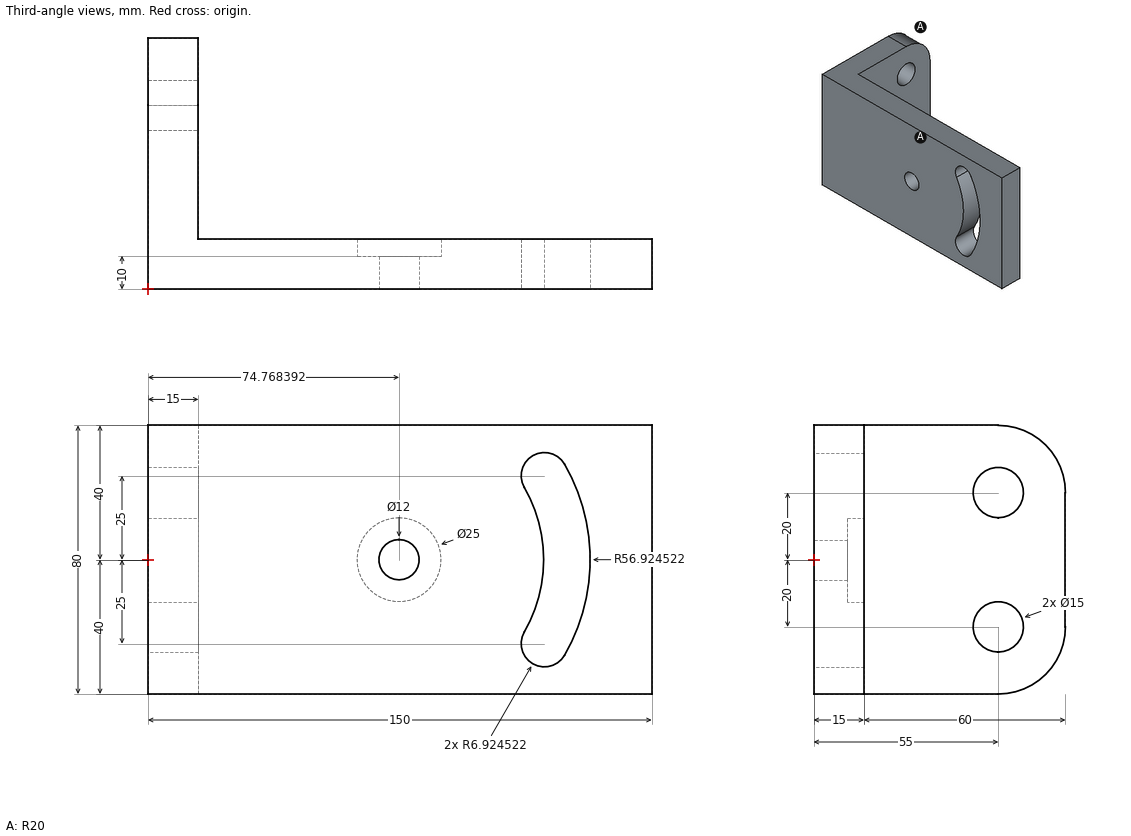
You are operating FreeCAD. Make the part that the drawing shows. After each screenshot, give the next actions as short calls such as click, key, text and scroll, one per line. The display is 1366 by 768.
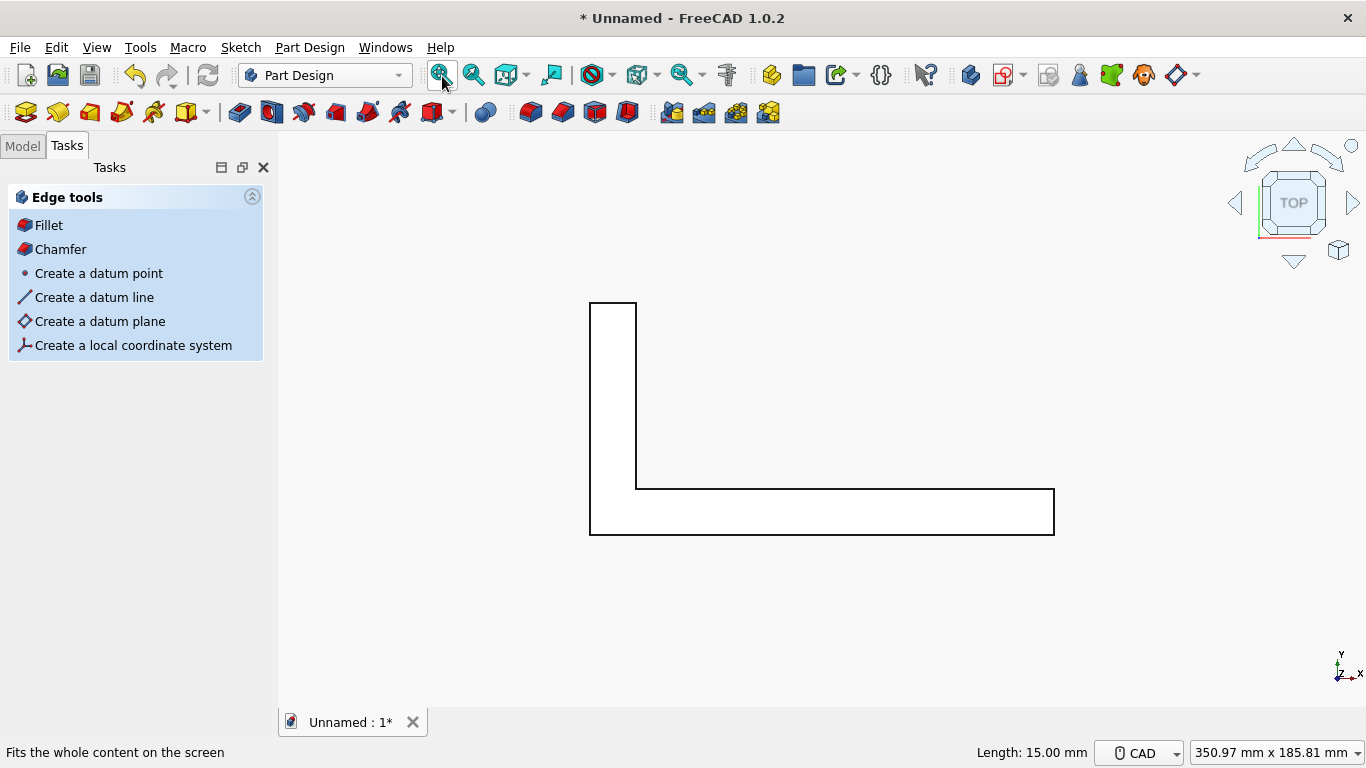
click(613, 302, ctrl)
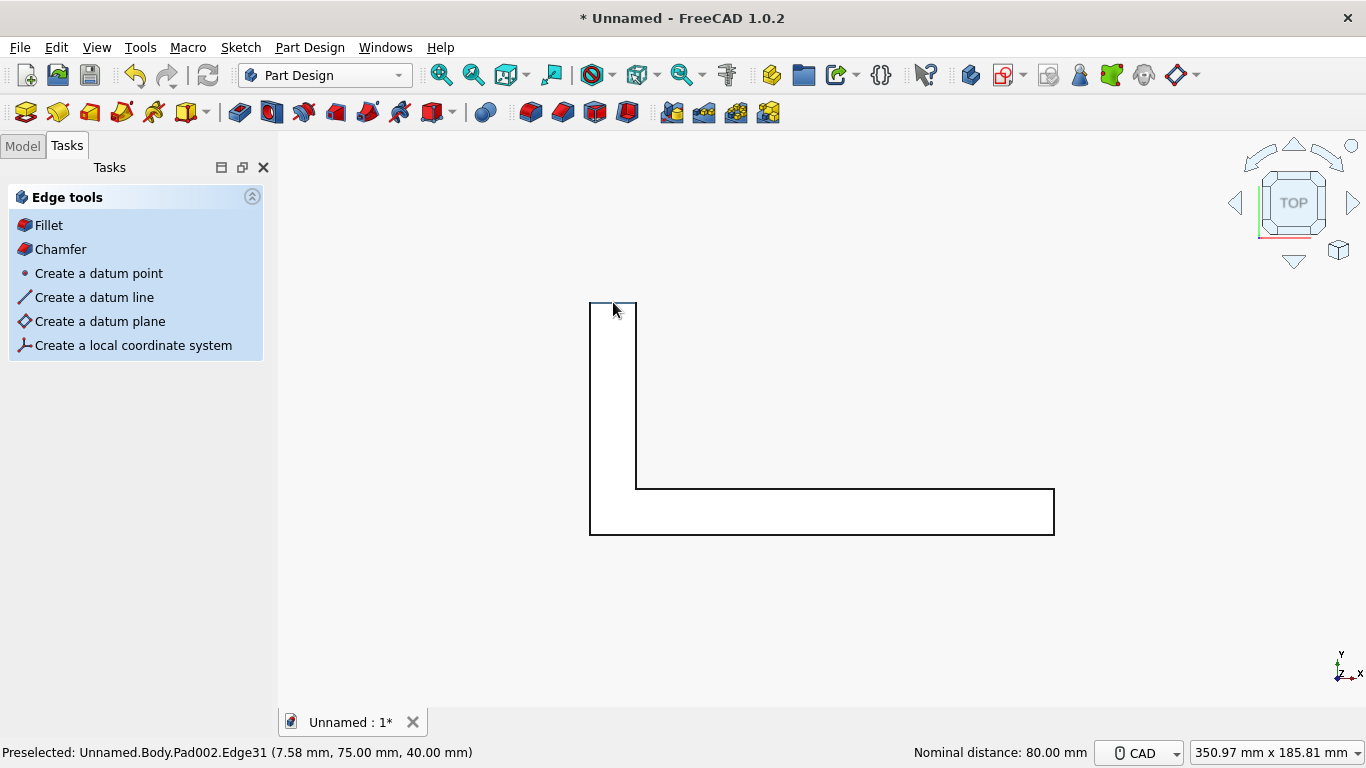
click(532, 112)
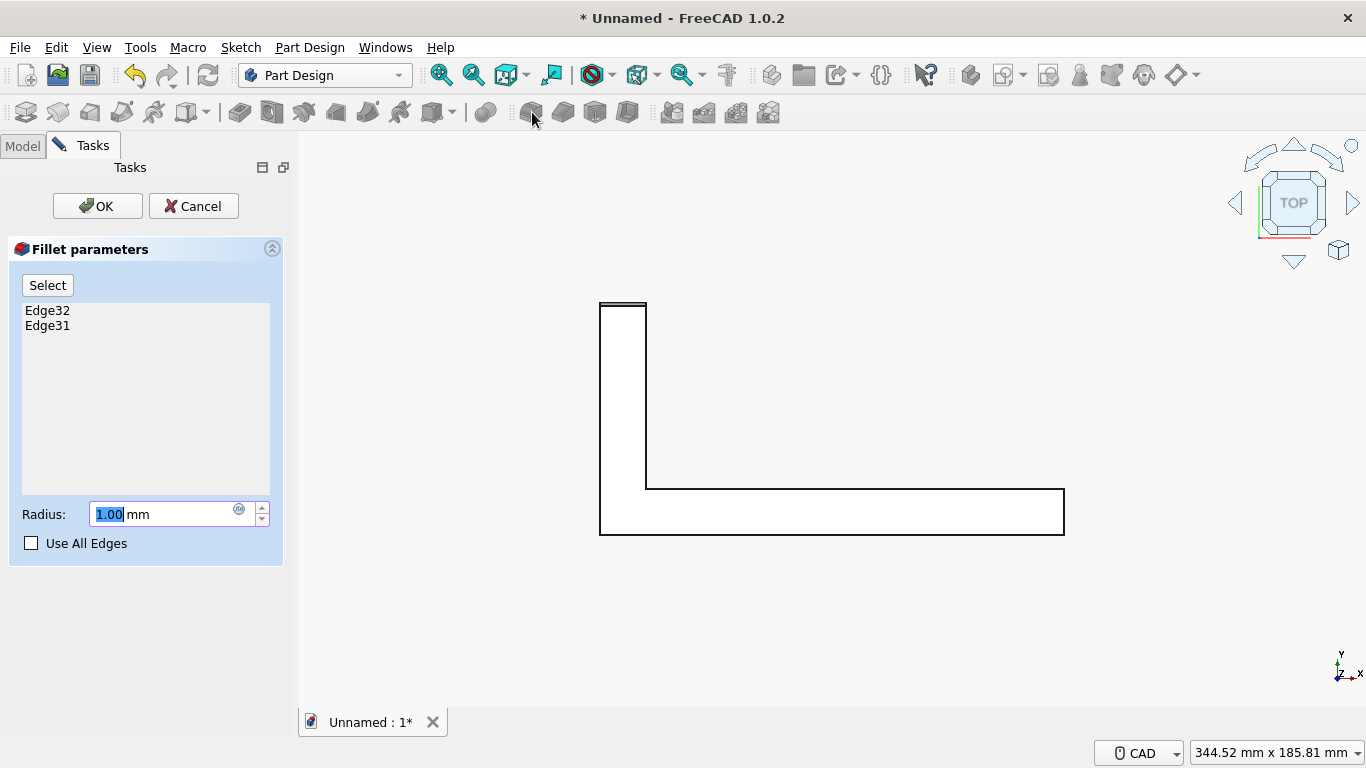
text(20)
key(Tab)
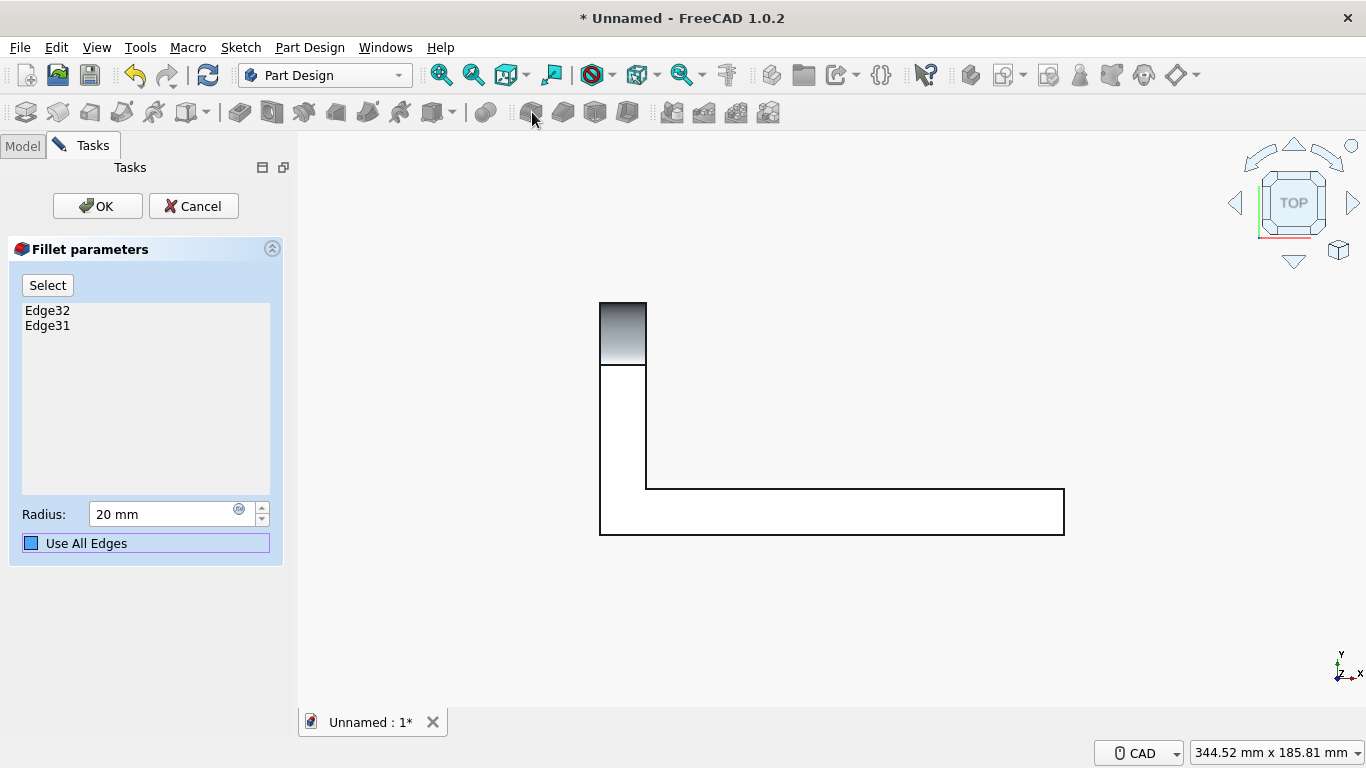
click(98, 206)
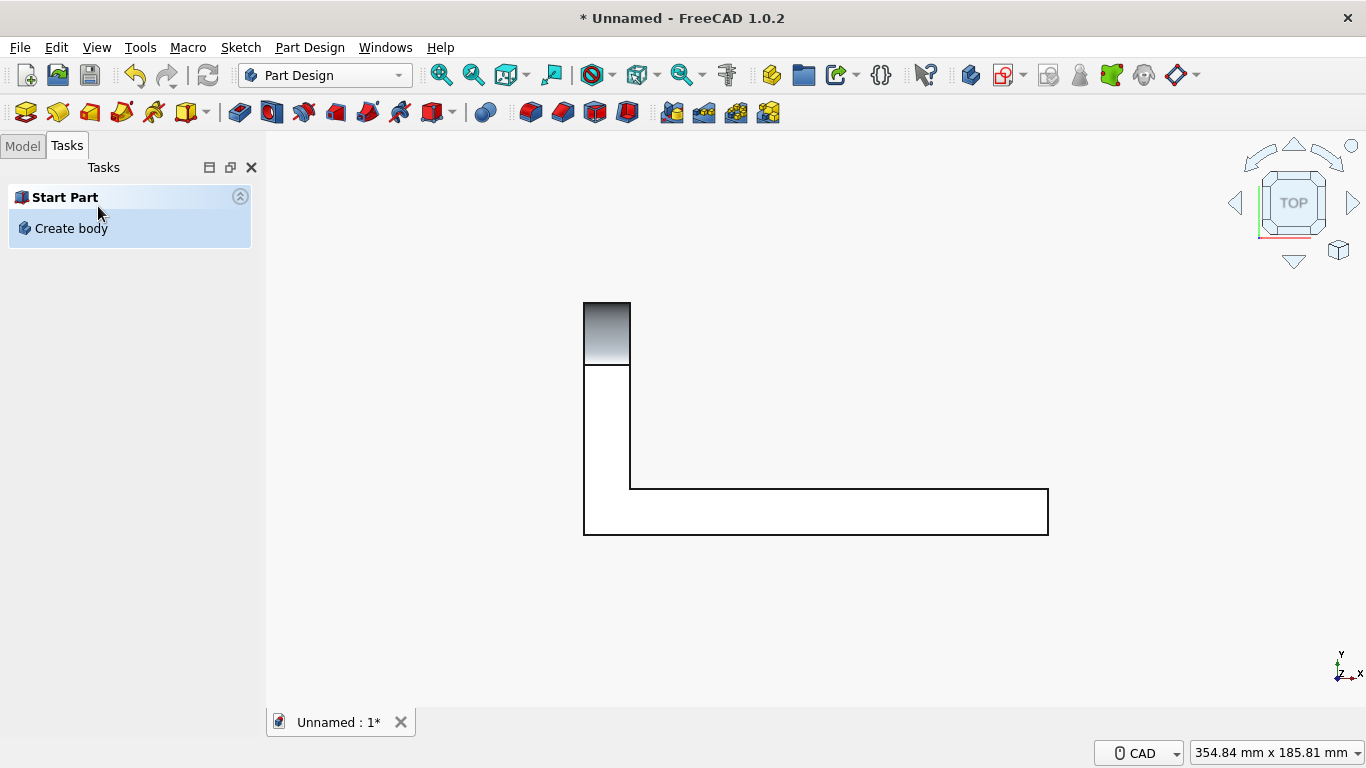
key(v)
key(f)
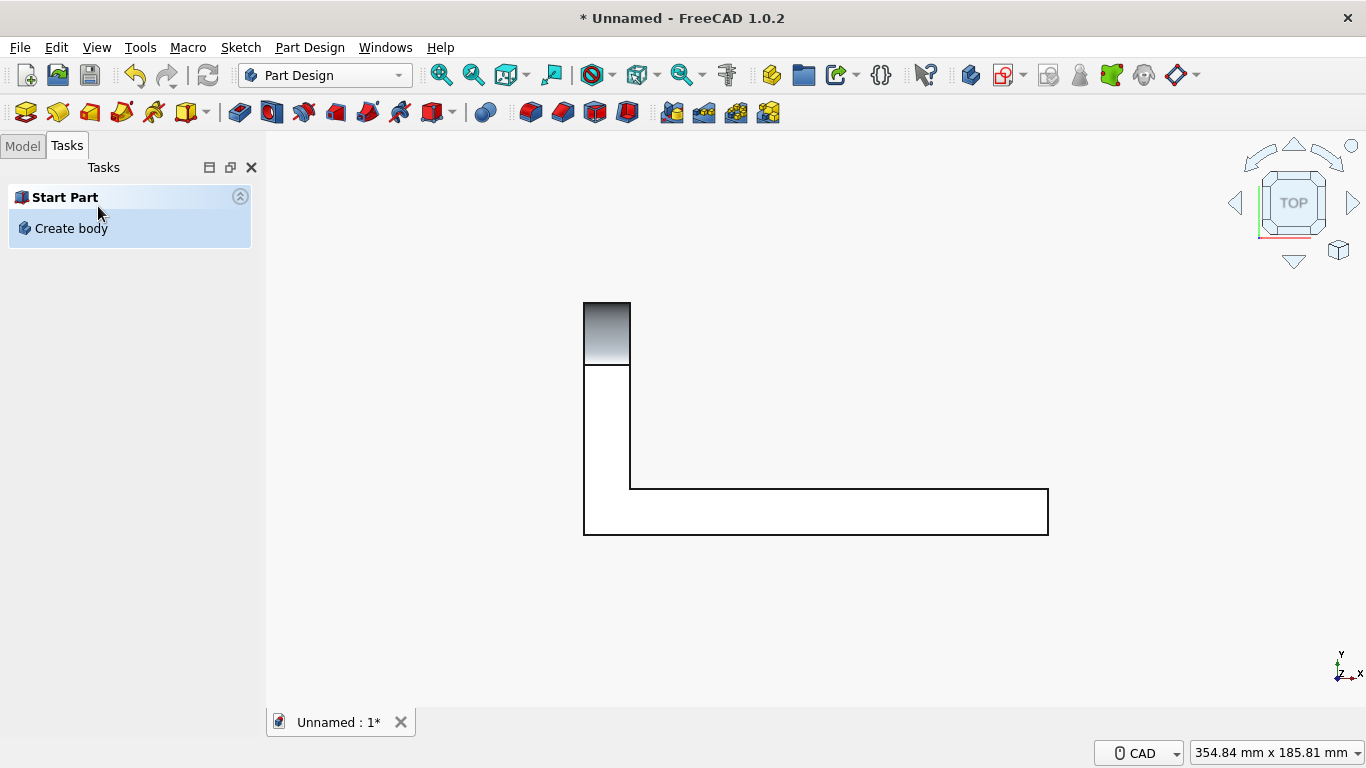
key(0)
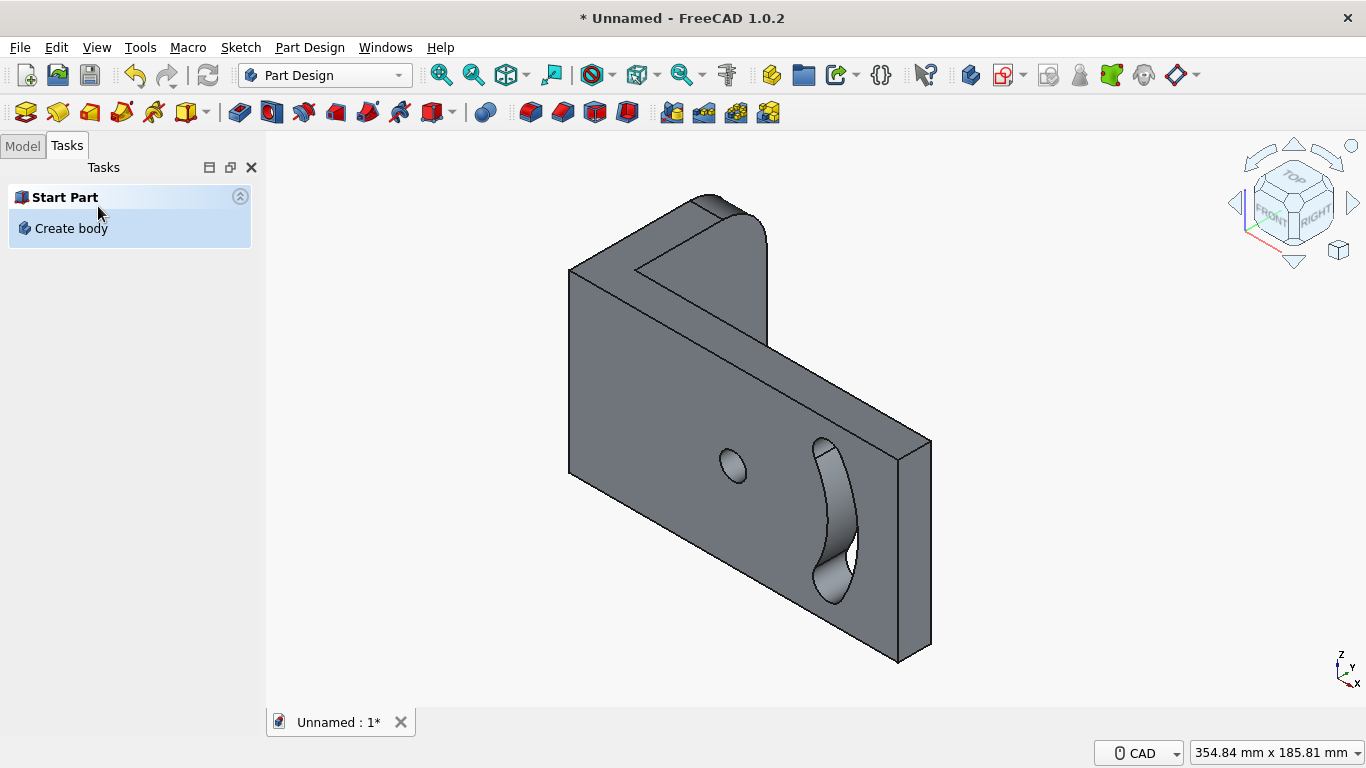
key(3)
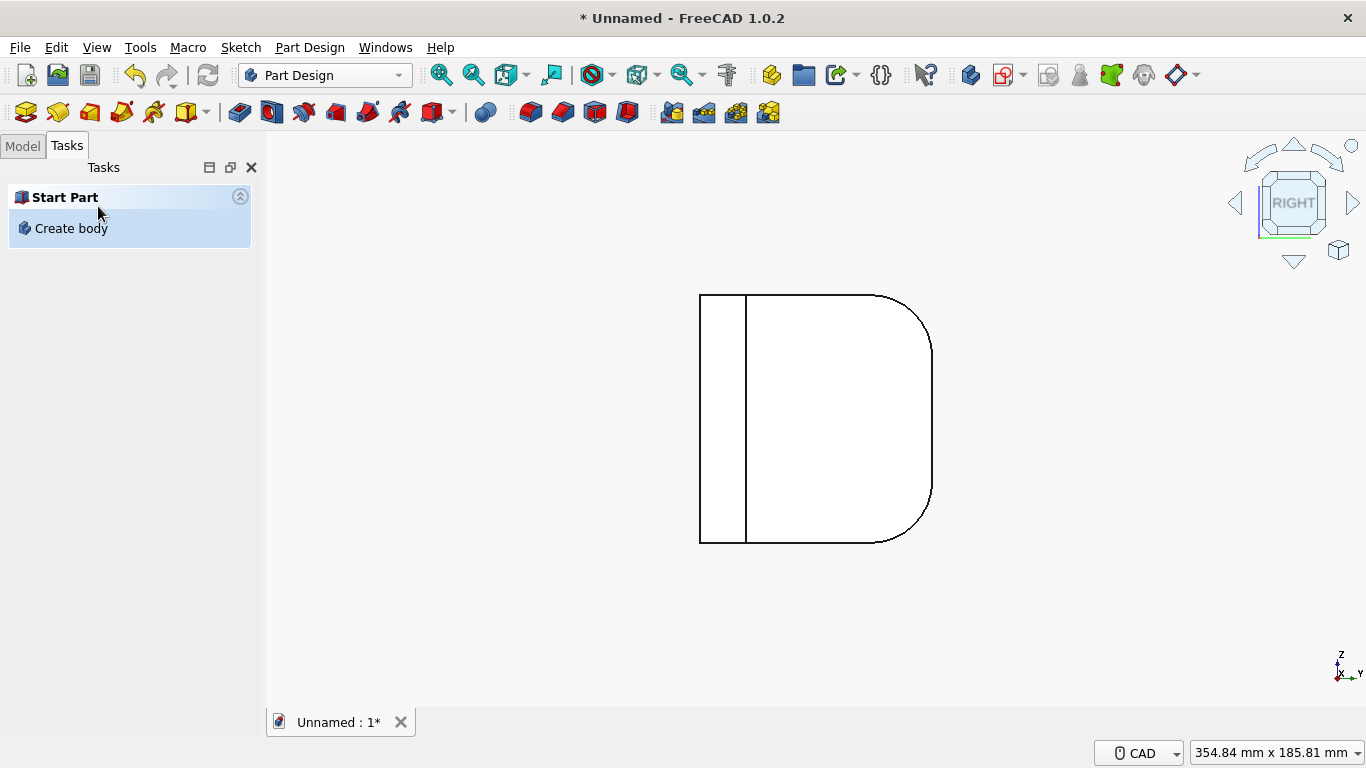
click(442, 76)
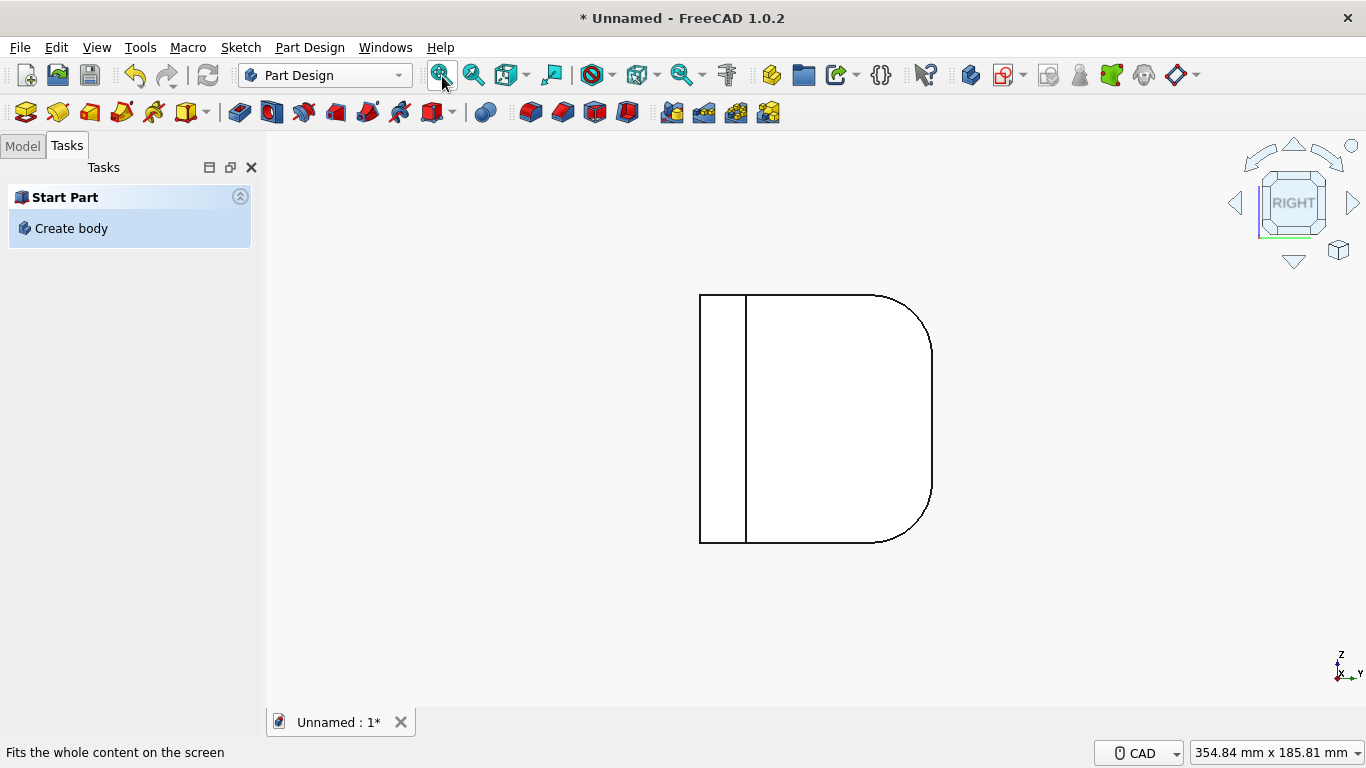
click(839, 418)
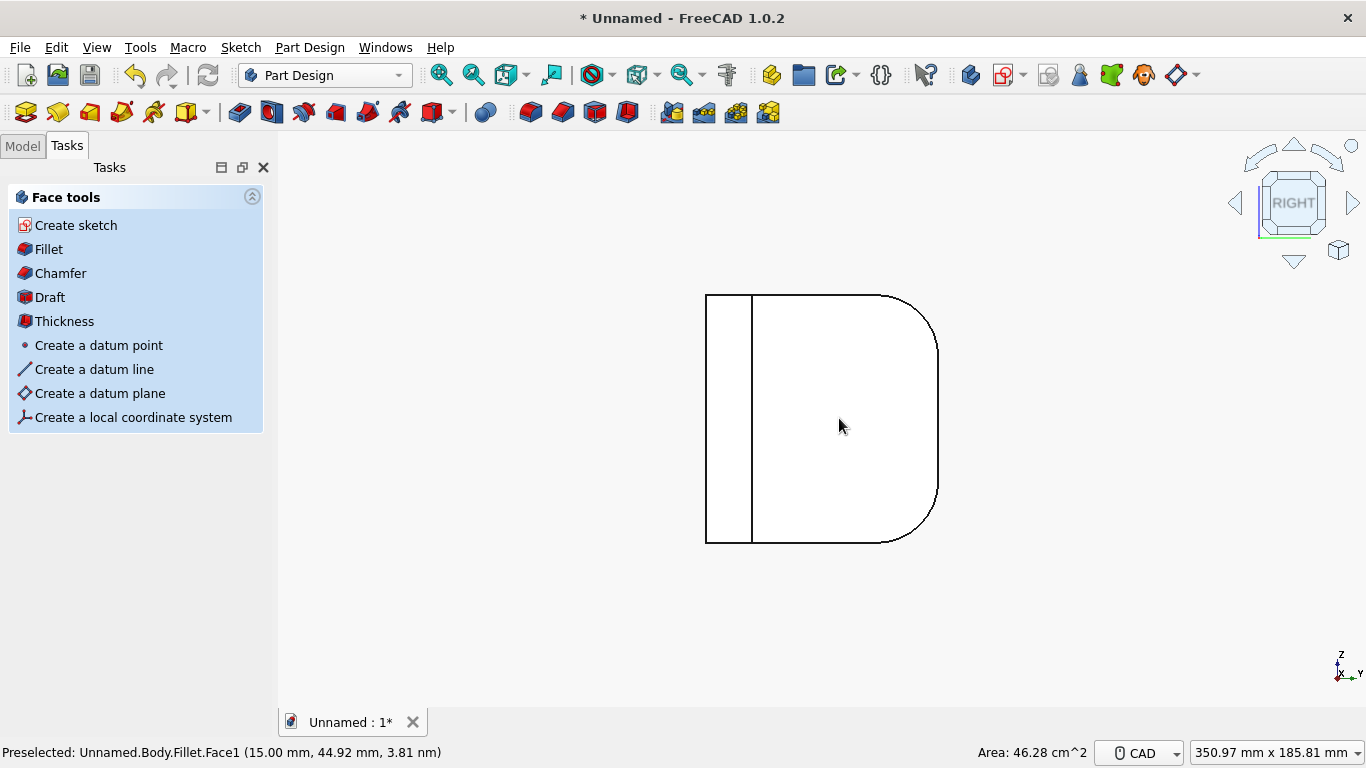
click(1004, 76)